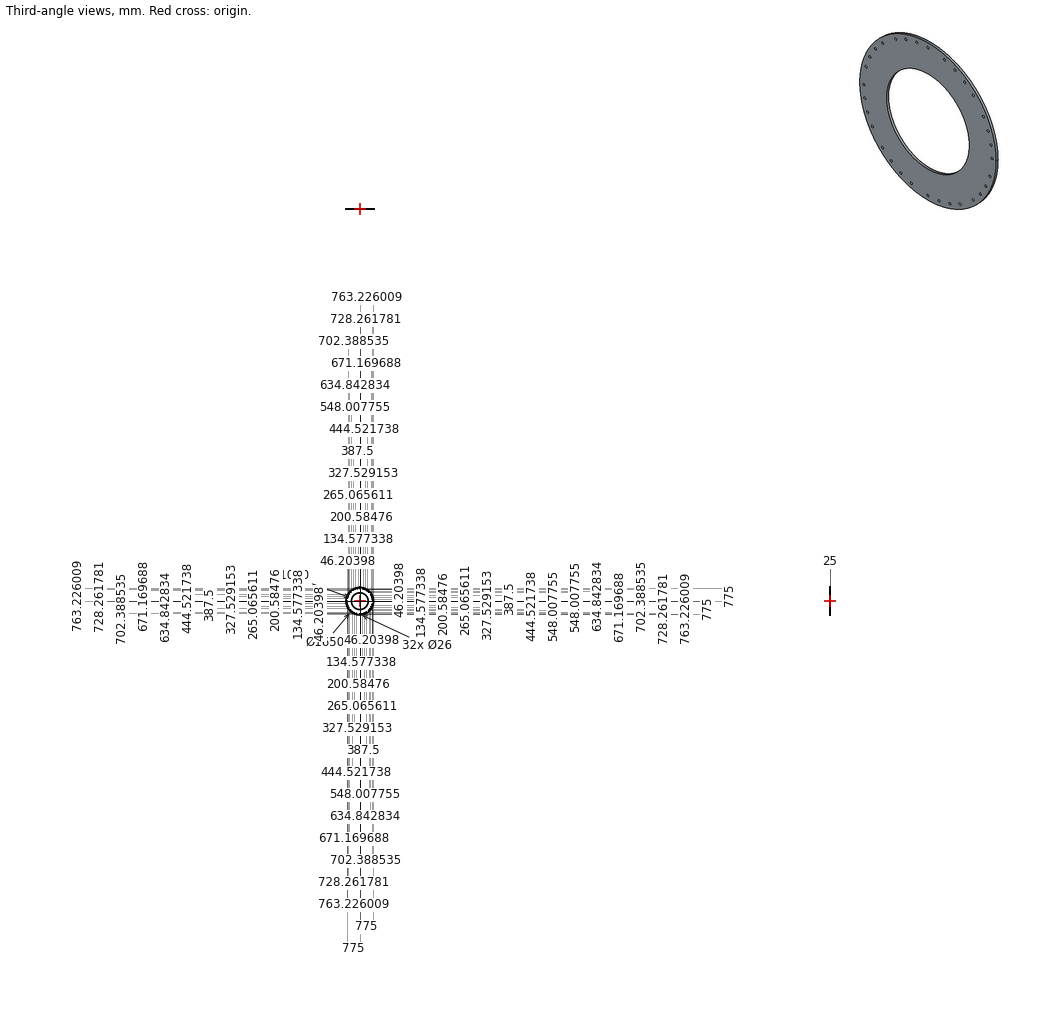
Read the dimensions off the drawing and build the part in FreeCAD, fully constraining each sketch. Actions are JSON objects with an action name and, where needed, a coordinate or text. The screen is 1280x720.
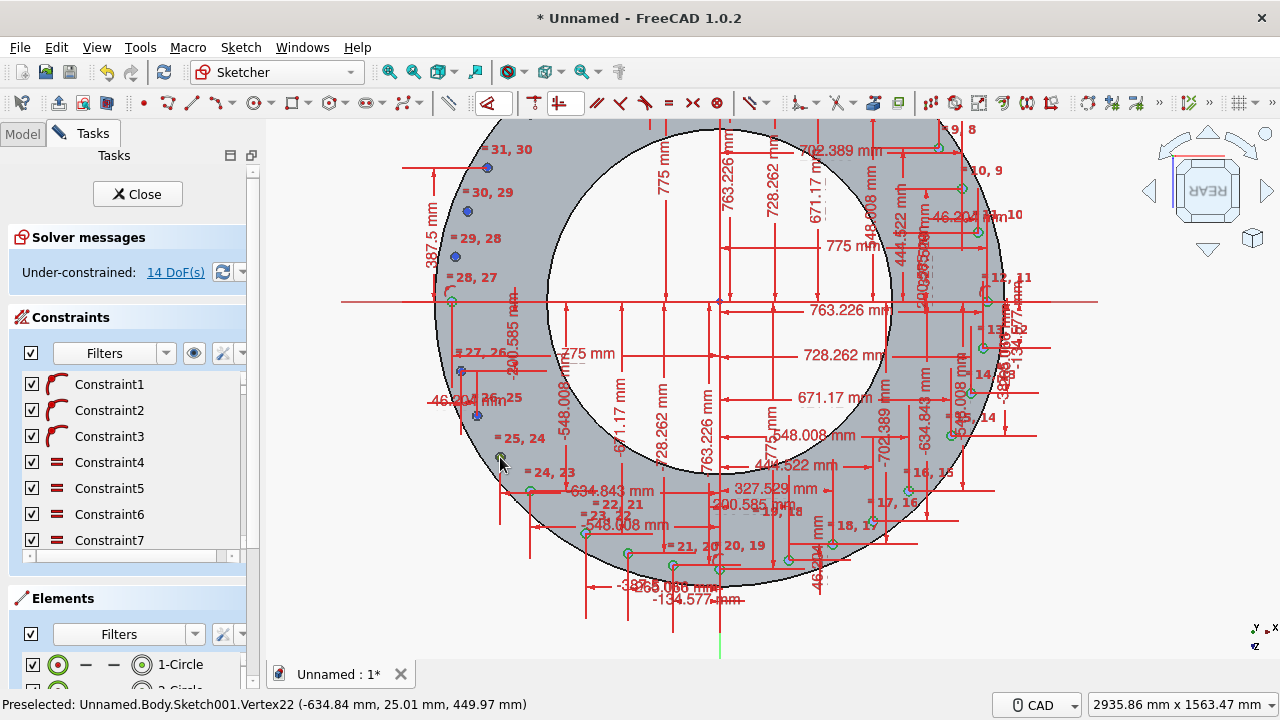
{"action": "key", "text": "i"}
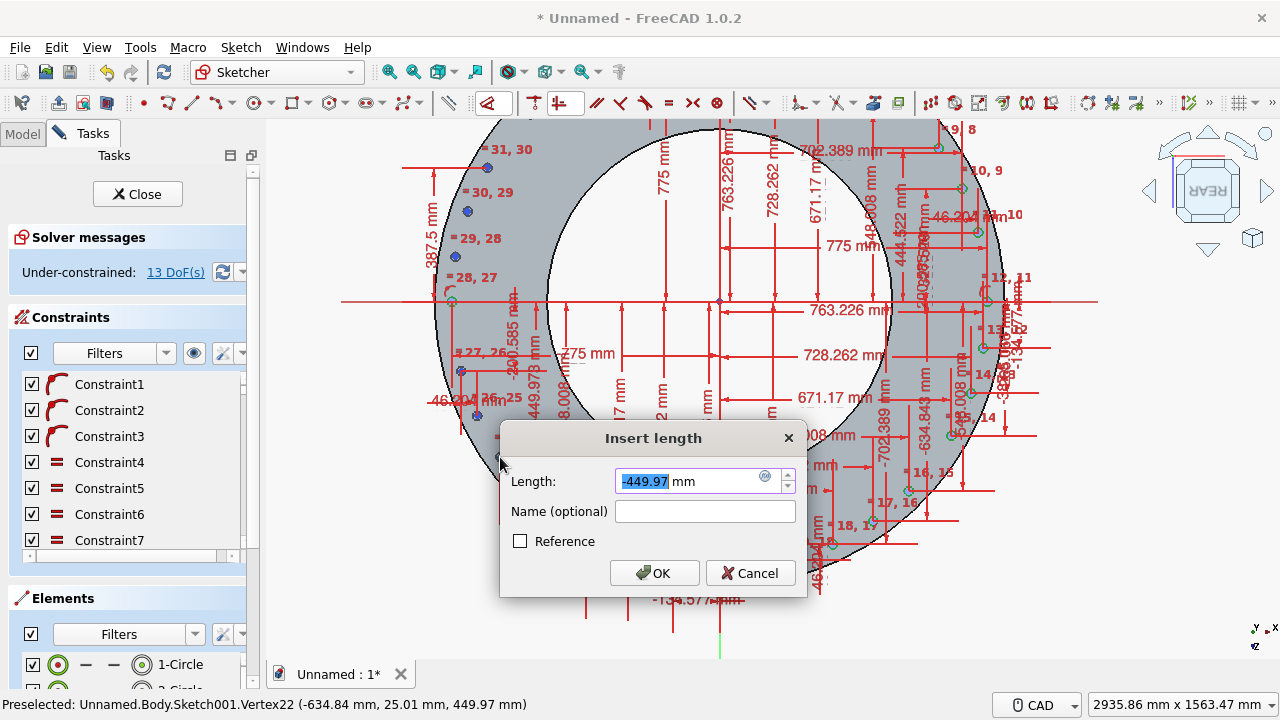
{"action": "type", "text": "-444.521738"}
{"action": "key", "text": "Return"}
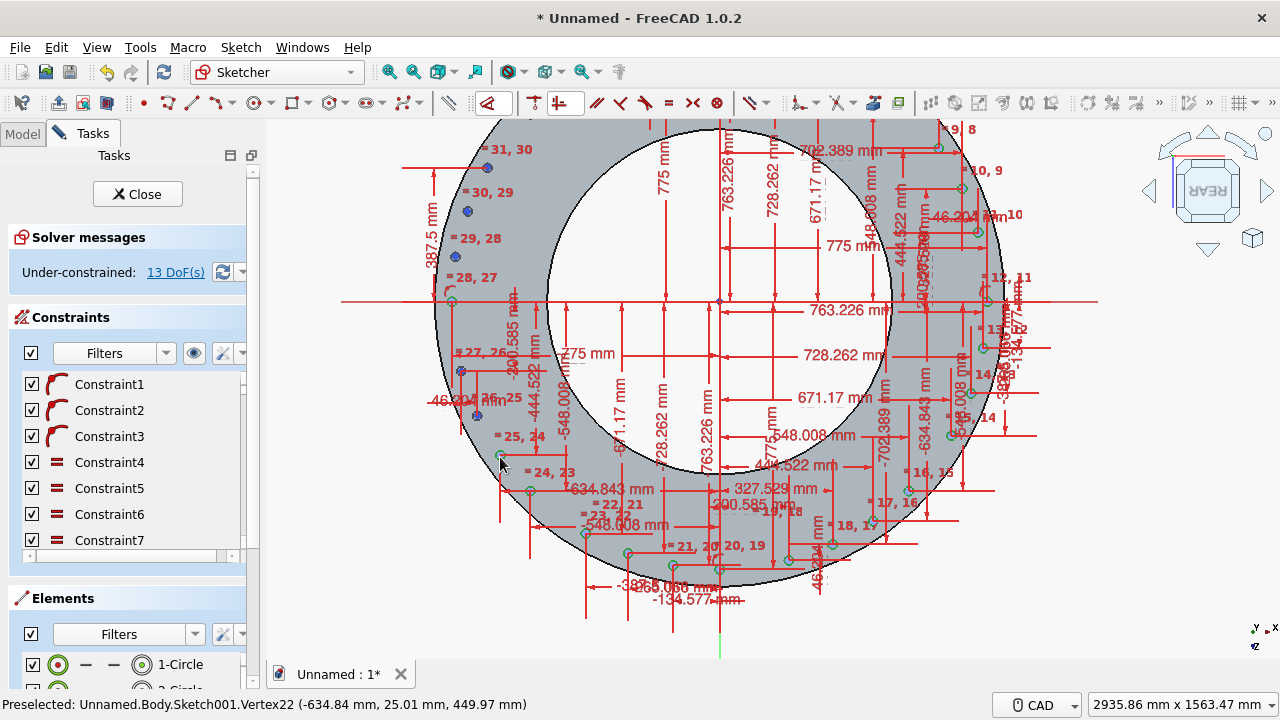
{"action": "left_click", "coordinate": [477, 416]}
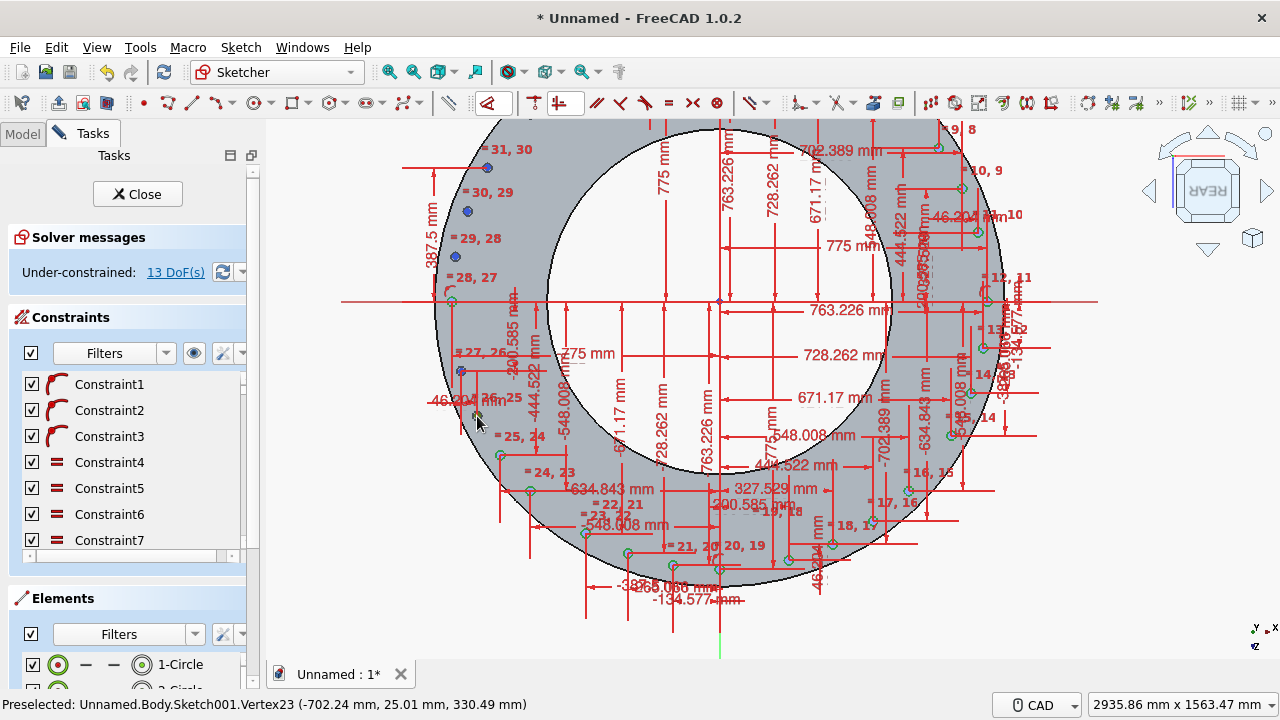
{"action": "key", "text": "l"}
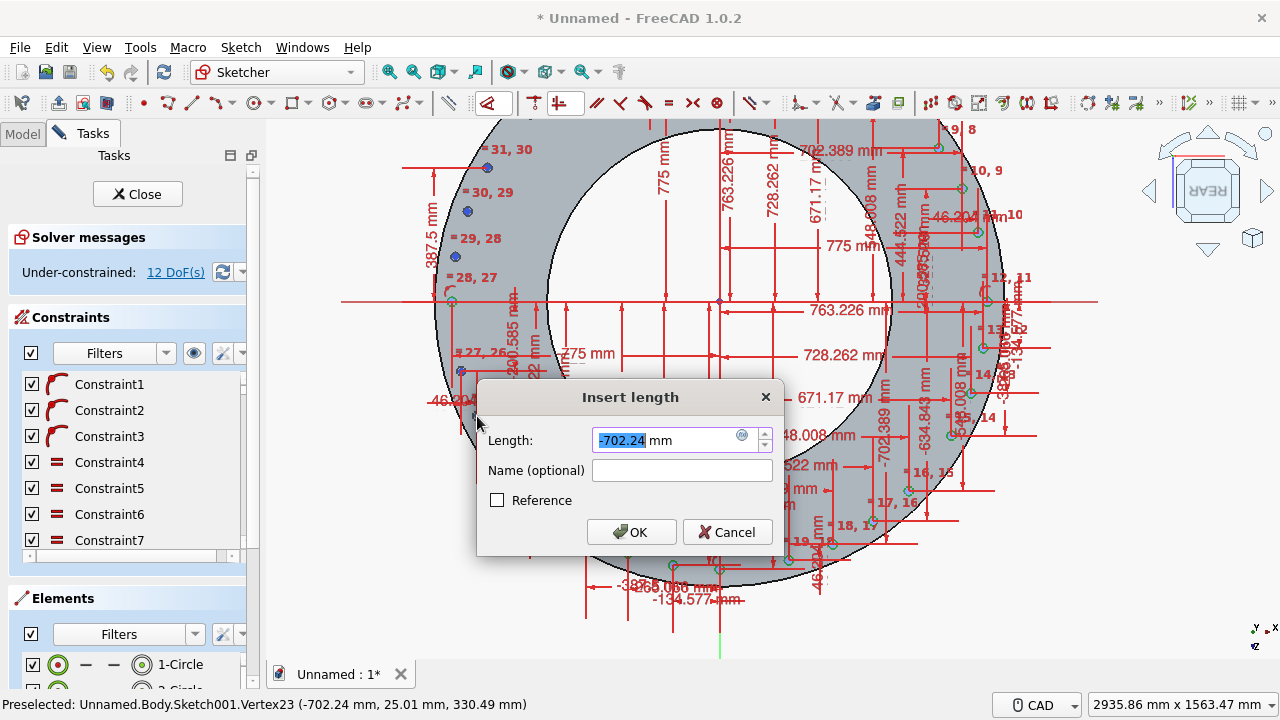
{"action": "type", "text": "-702.388535"}
{"action": "key", "text": "Return"}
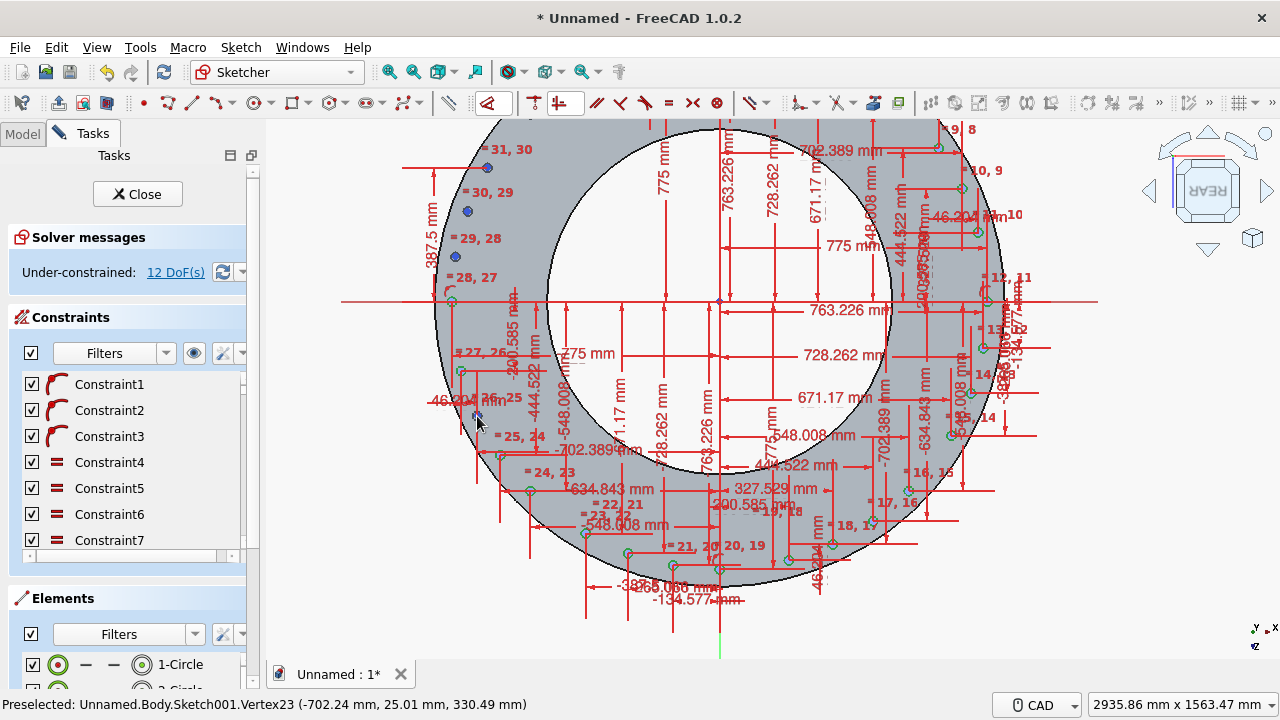
{"action": "left_click", "coordinate": [477, 416]}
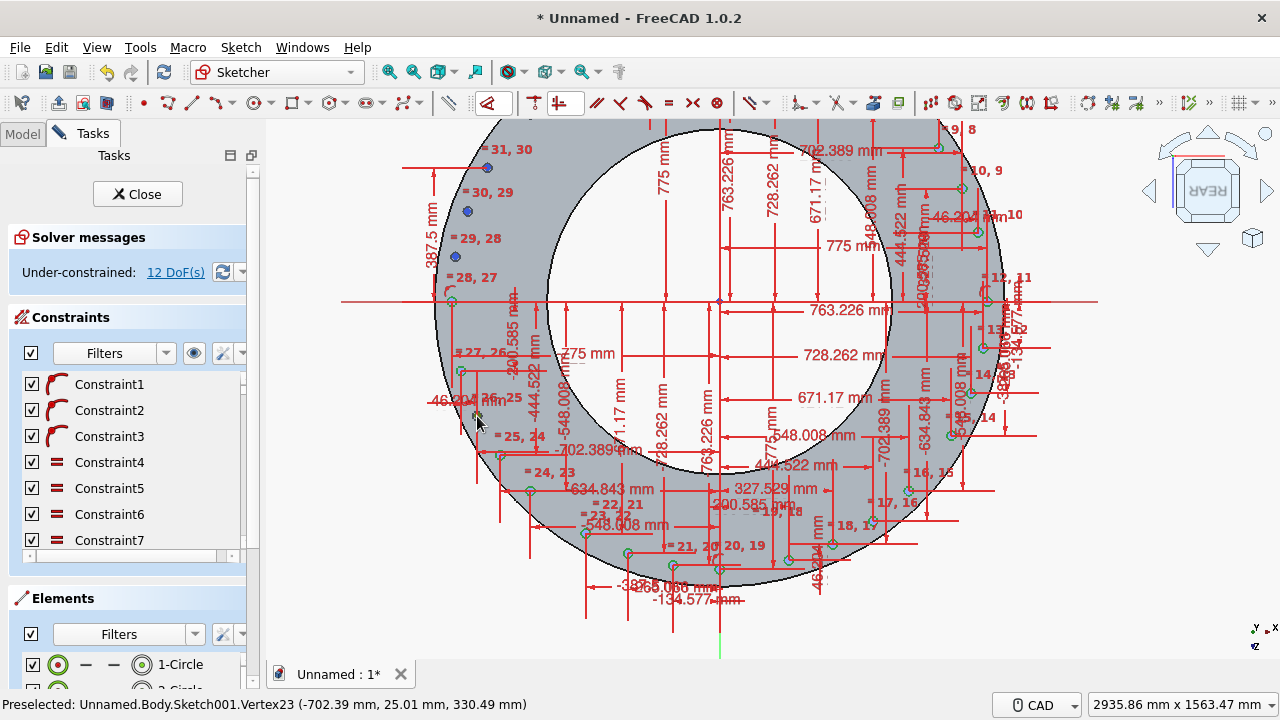
{"action": "key", "text": "i"}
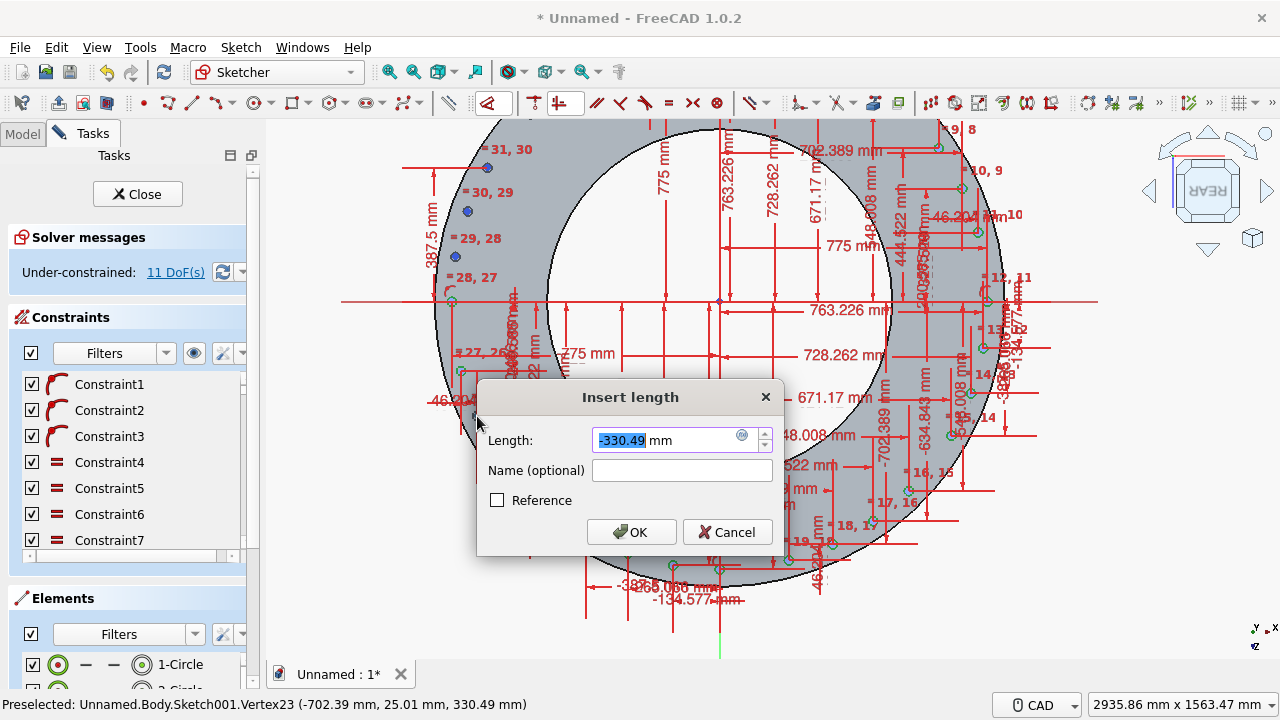
{"action": "type", "text": "-327.529153"}
{"action": "key", "text": "Return"}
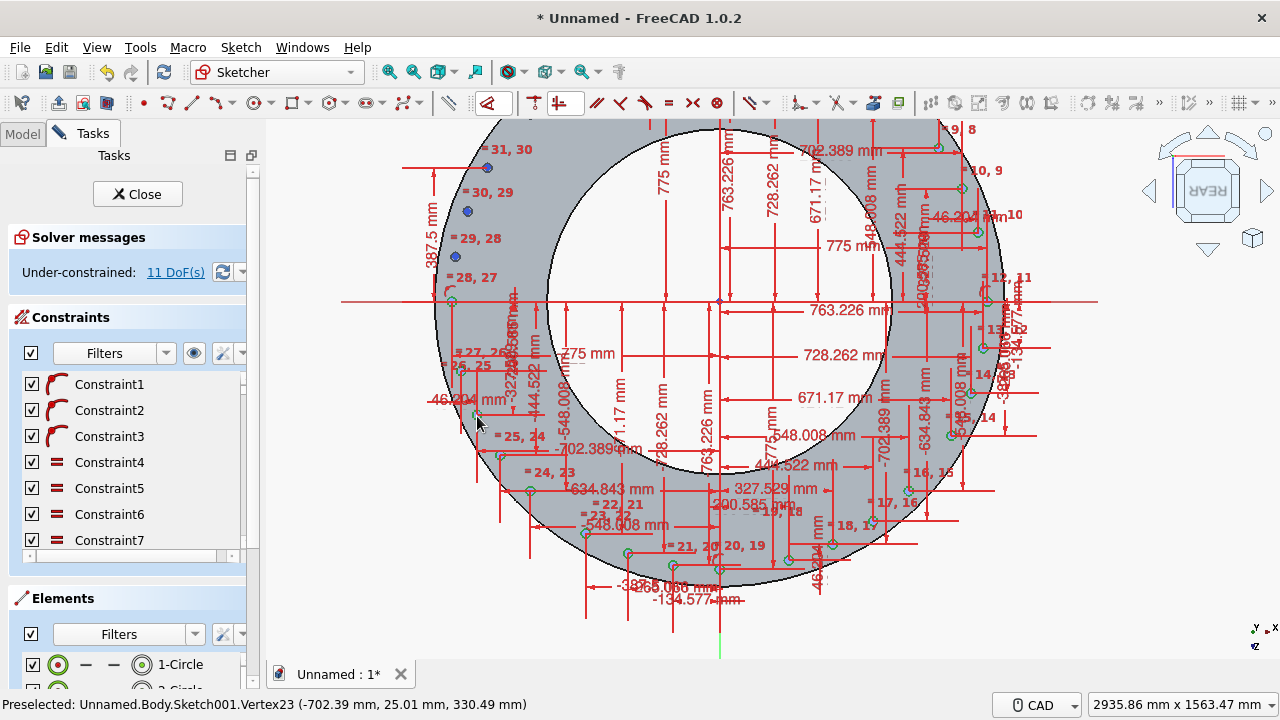
{"action": "left_click", "coordinate": [456, 257]}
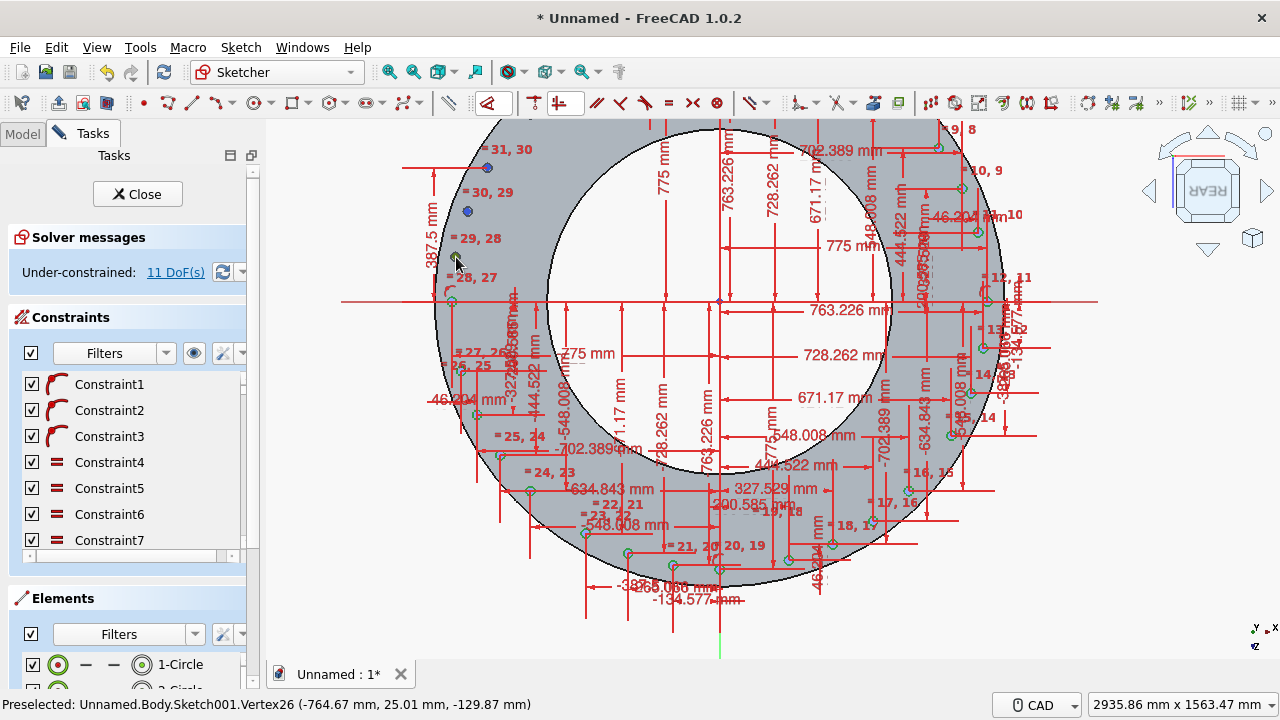
{"action": "key", "text": "l"}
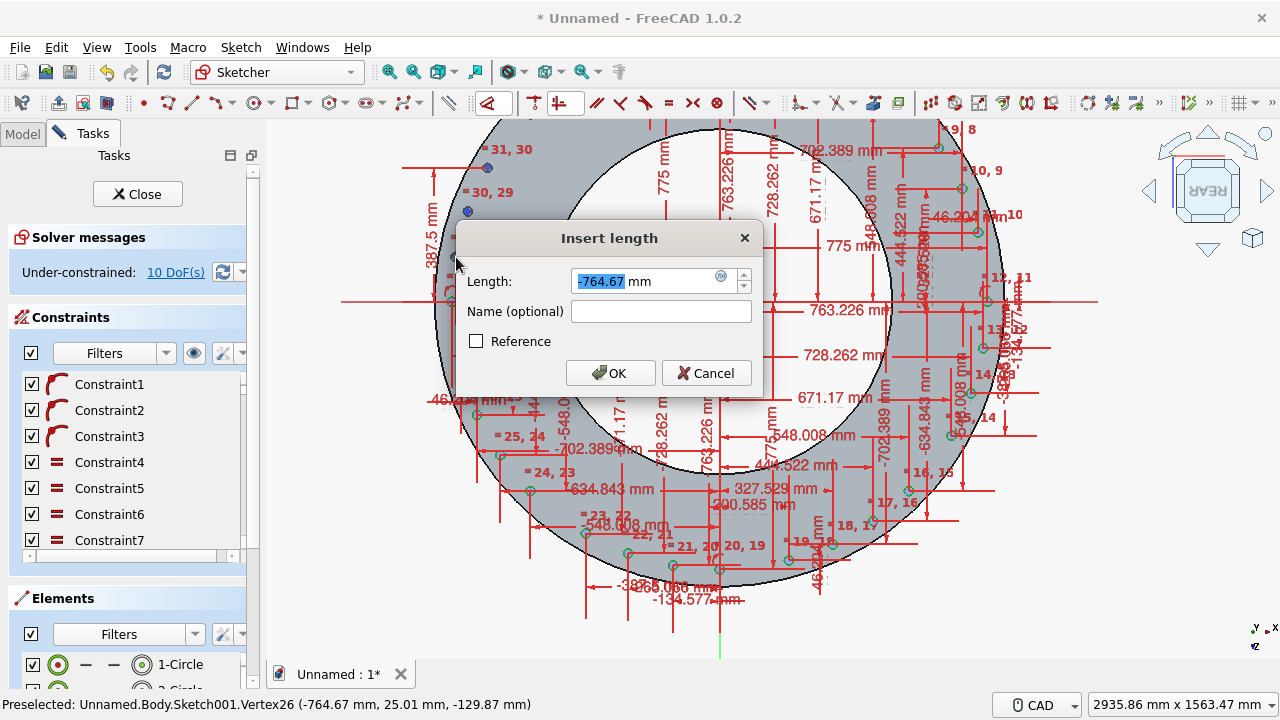
{"action": "type", "text": "-763.226009"}
{"action": "key", "text": "Return"}